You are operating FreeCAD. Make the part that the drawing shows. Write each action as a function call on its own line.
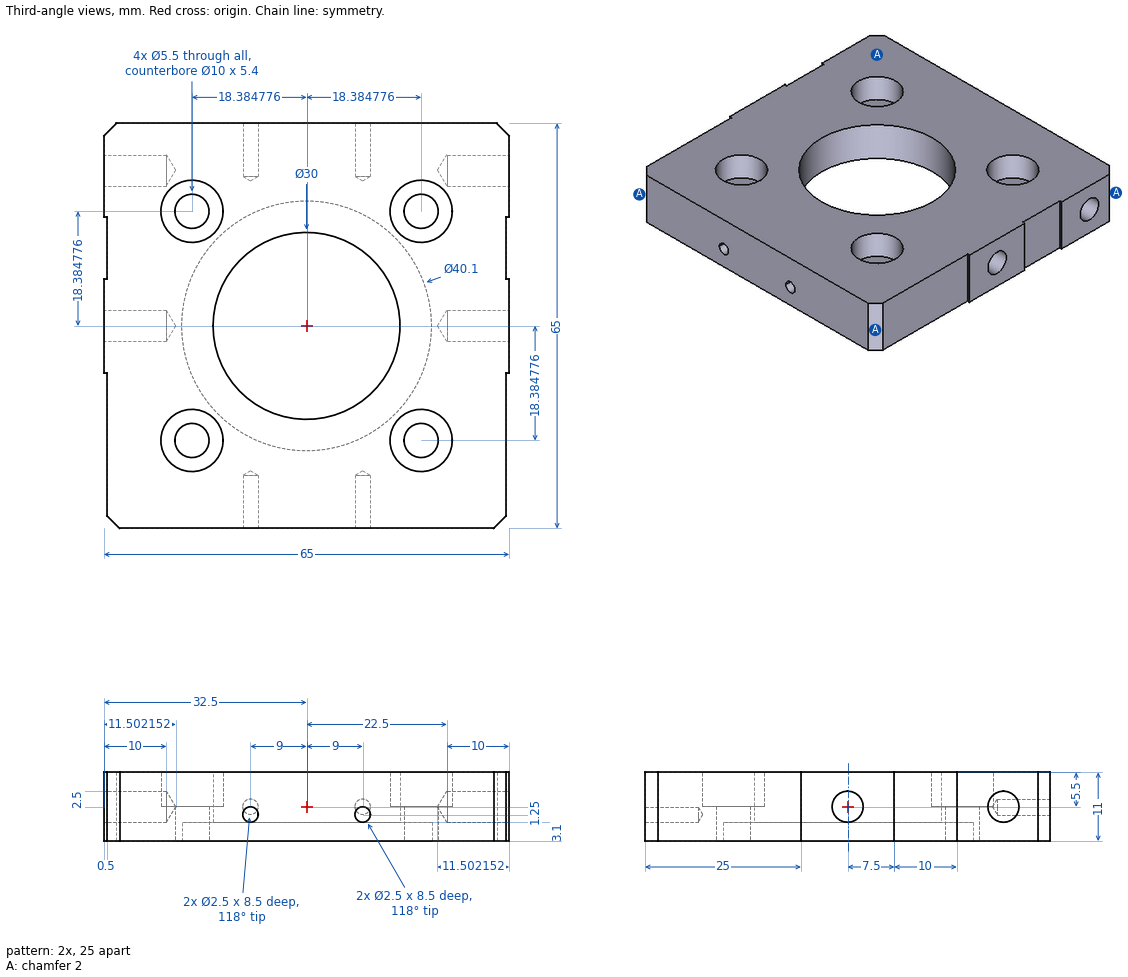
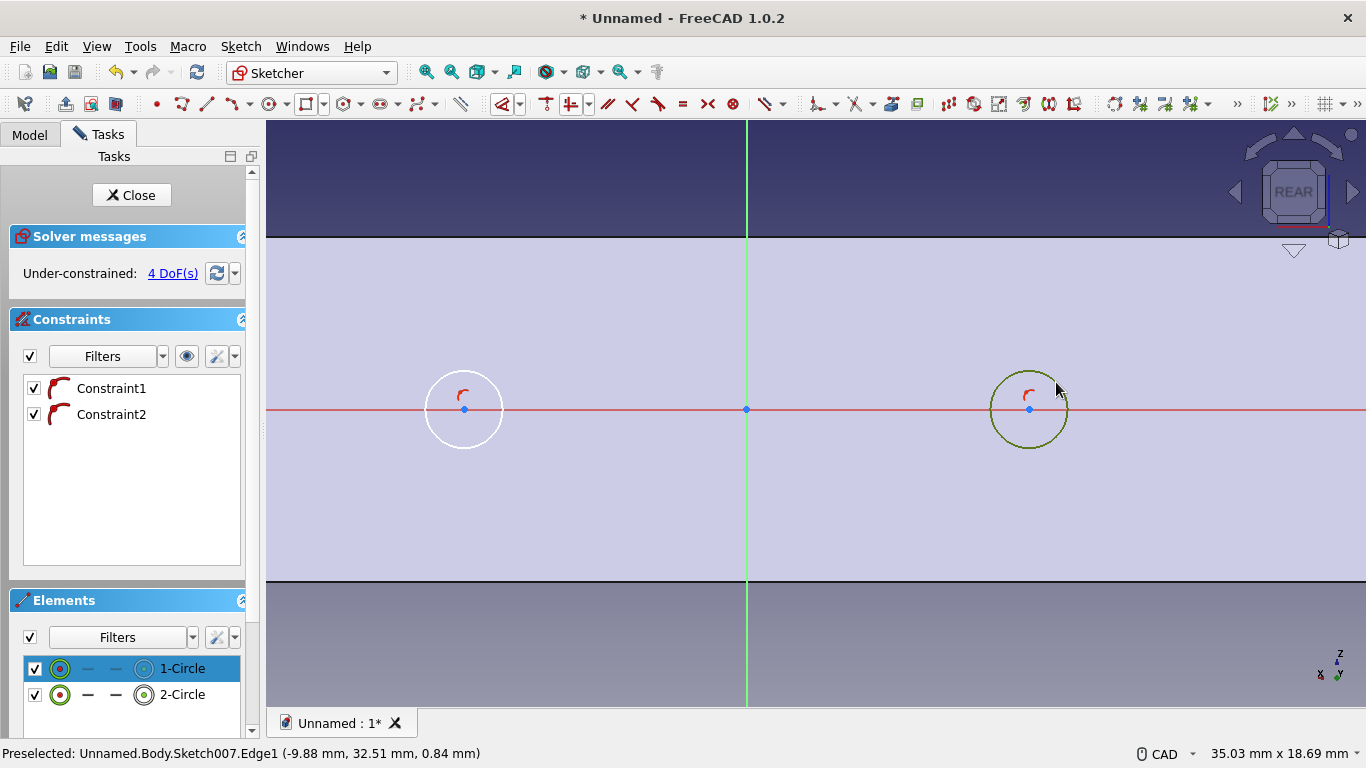
click(491, 382)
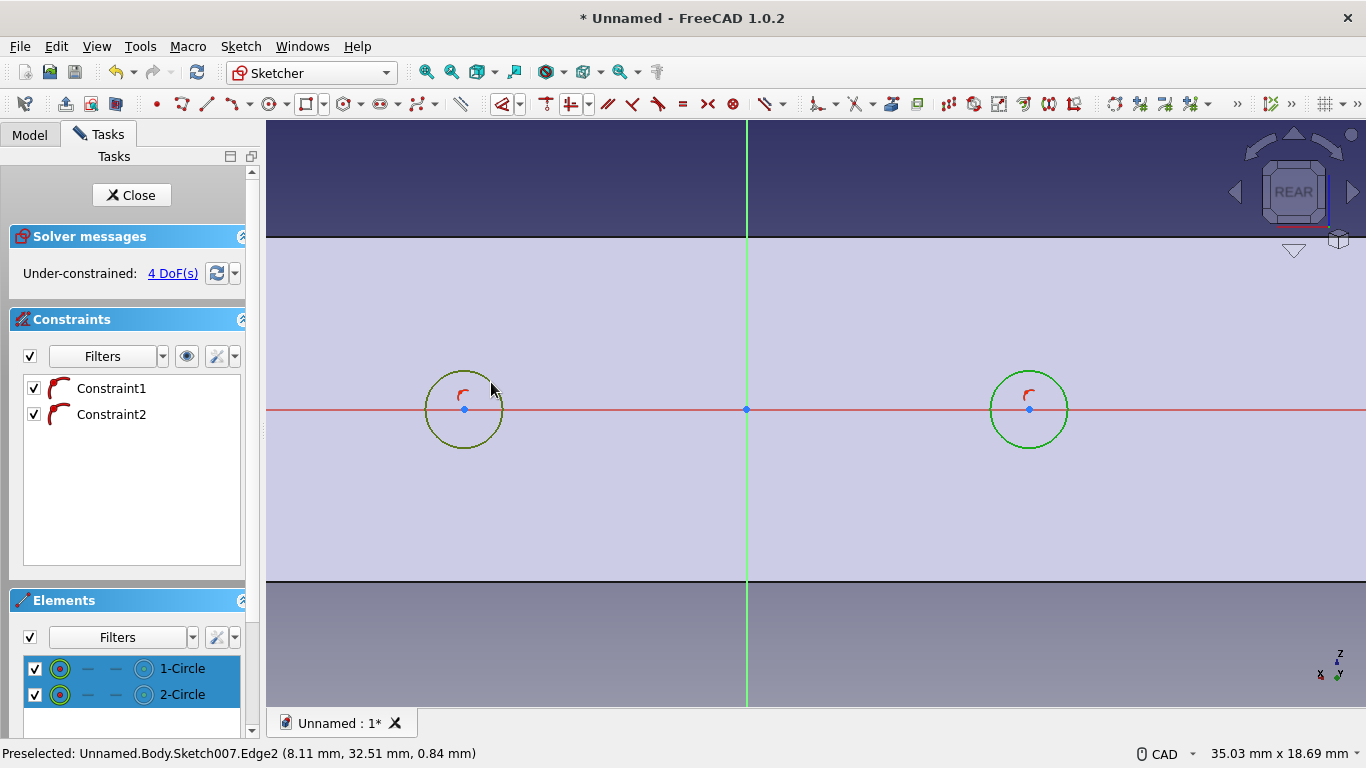
click(683, 104)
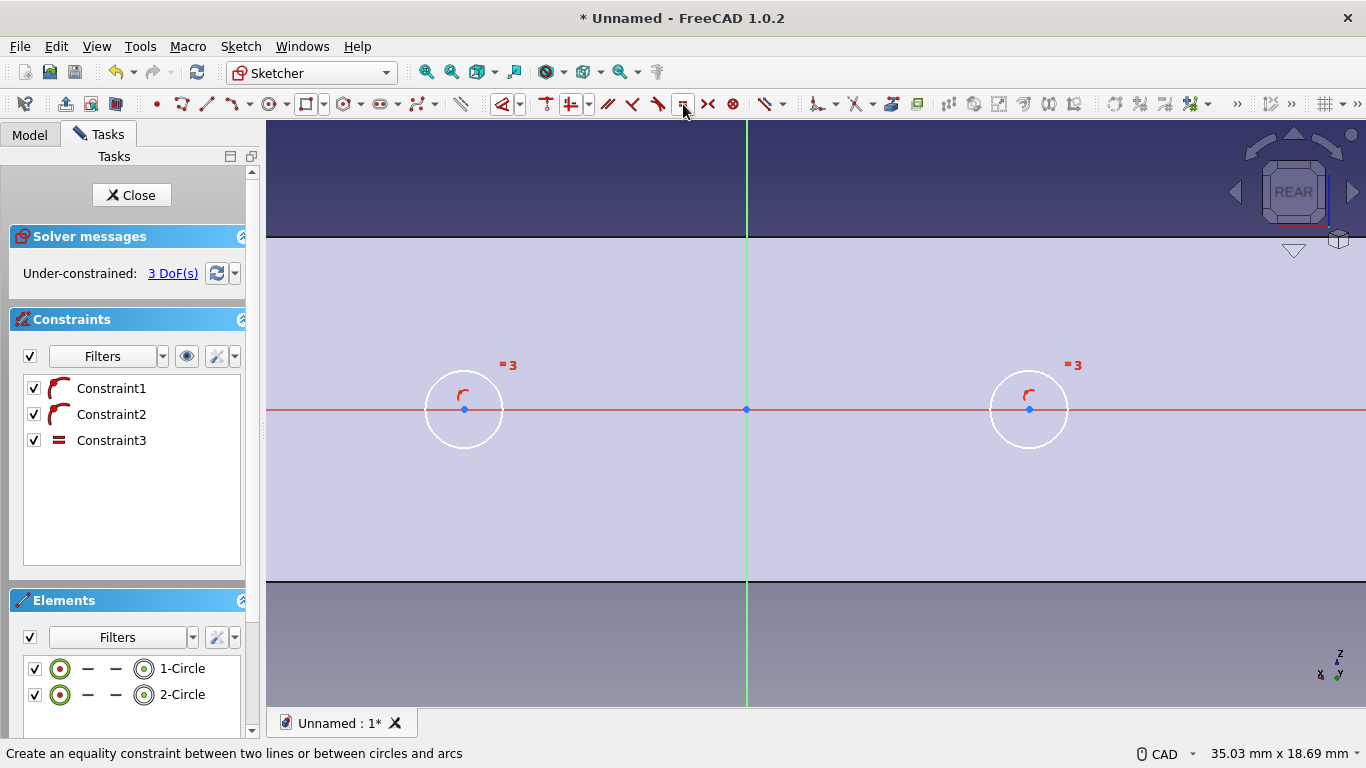
click(1056, 382)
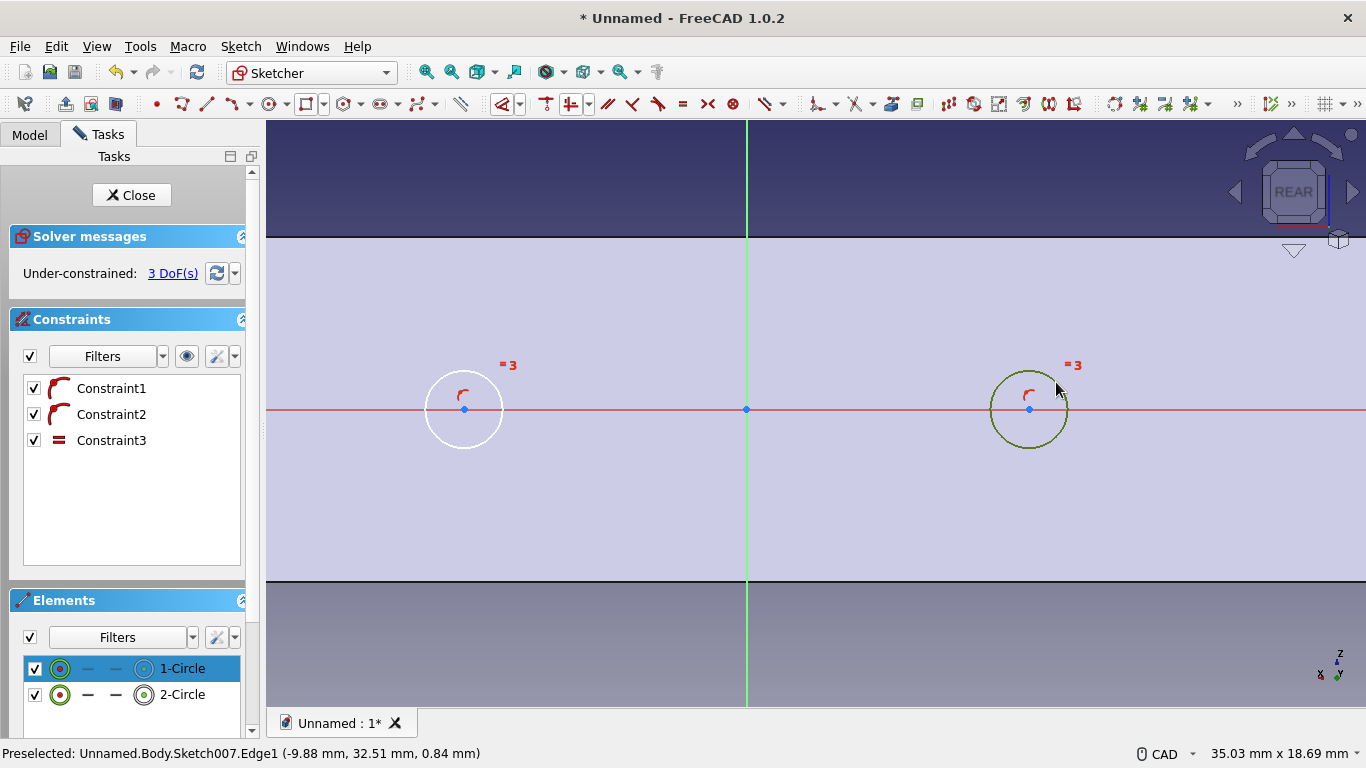
key(k)
key(o)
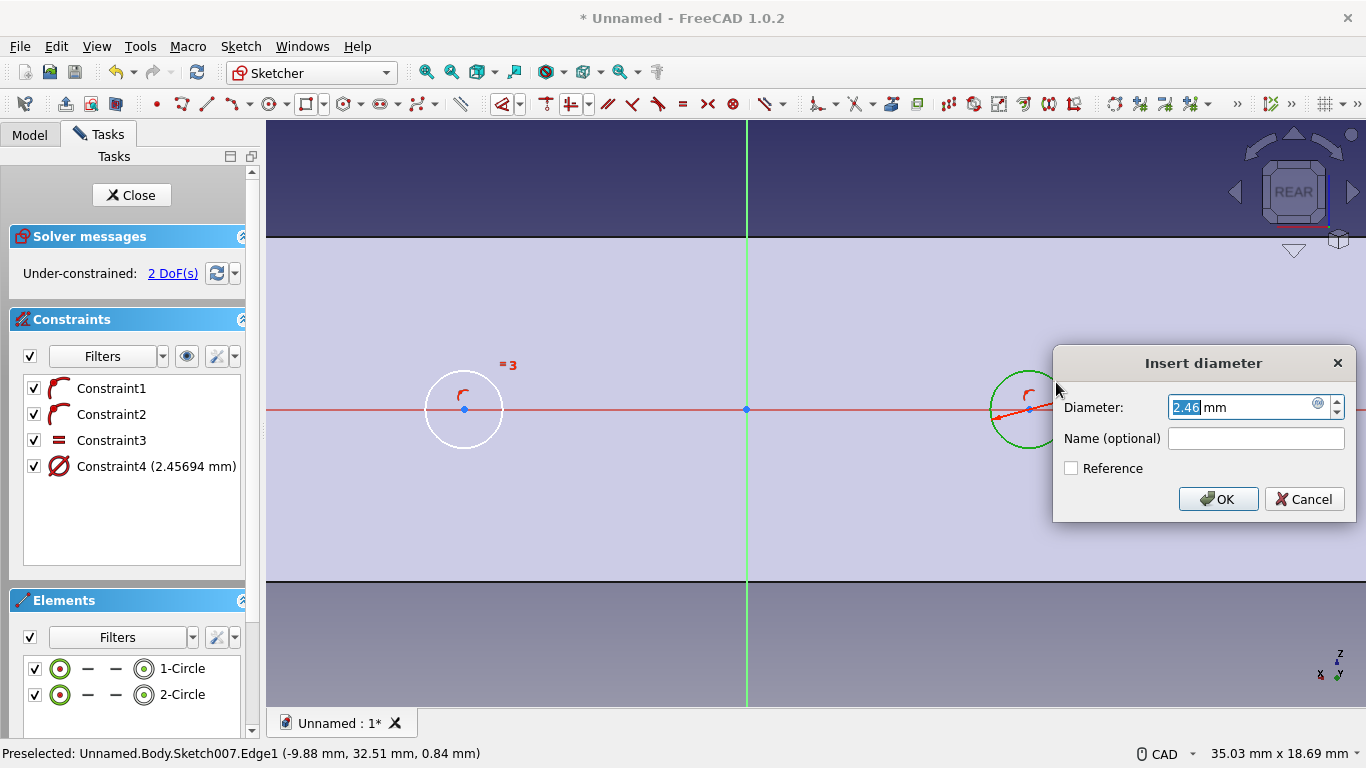
text(2.5)
key(Return)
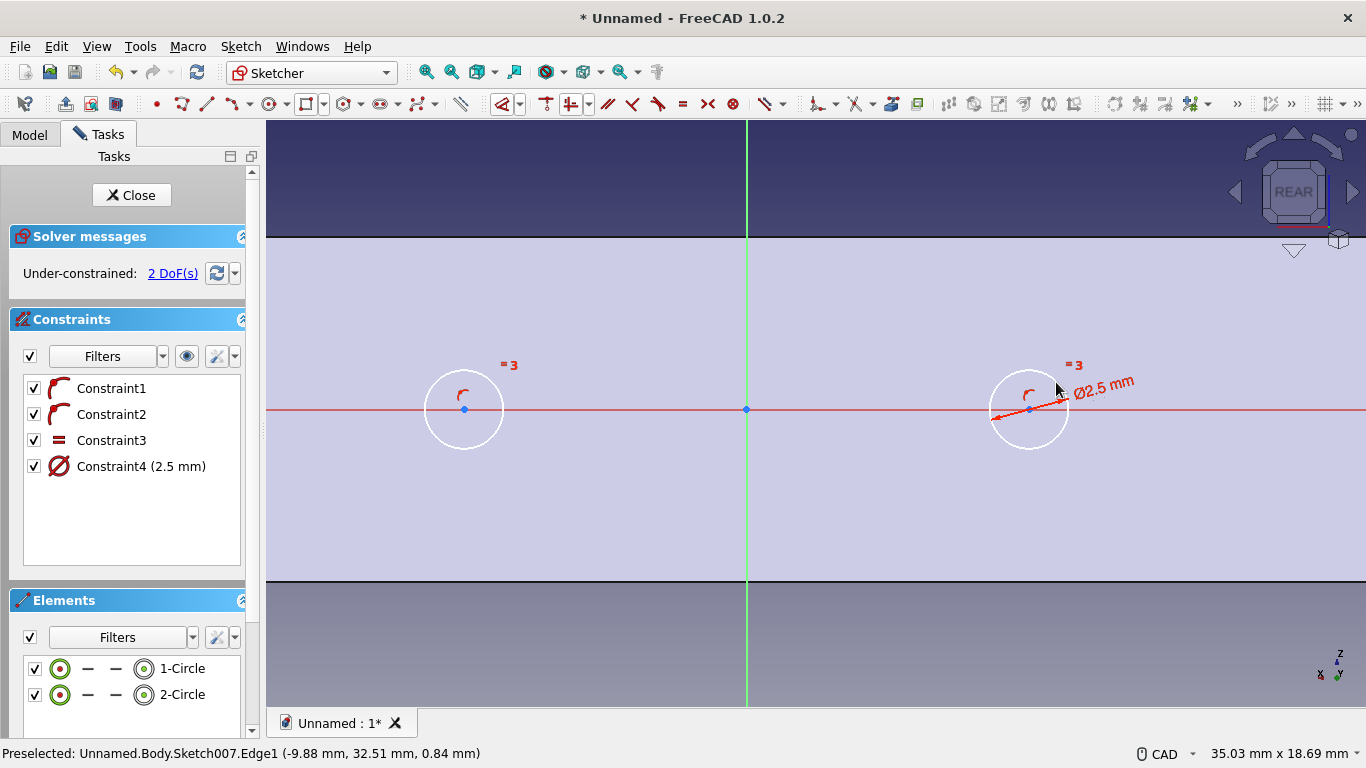
click(1029, 410)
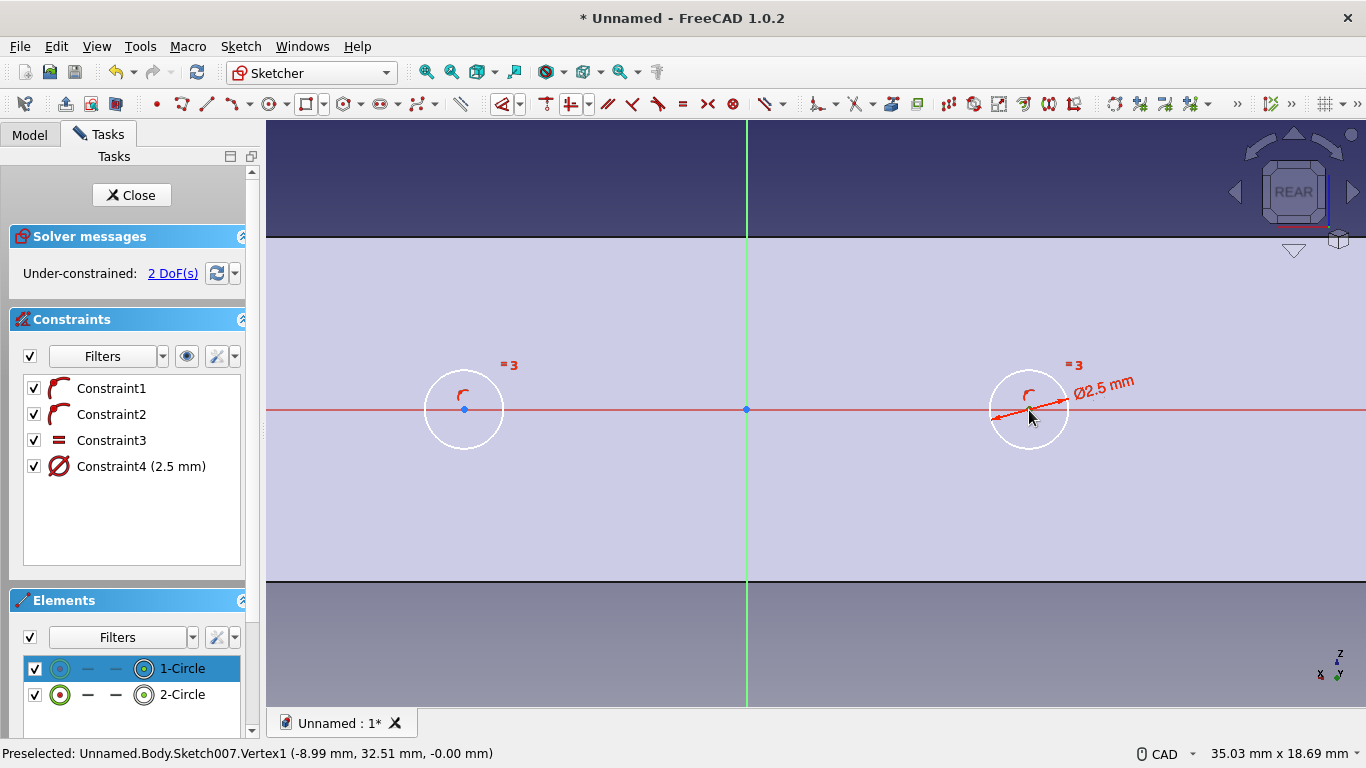
click(520, 104)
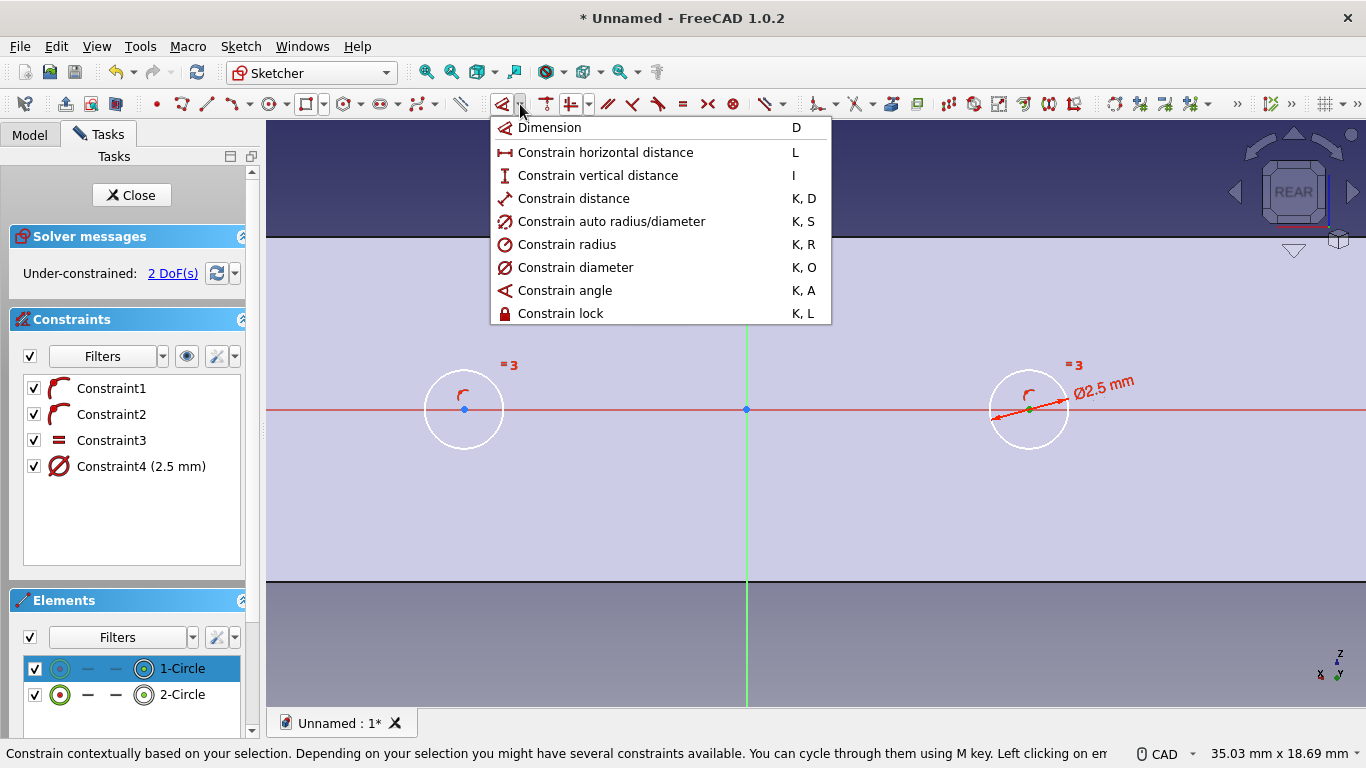
click(661, 152)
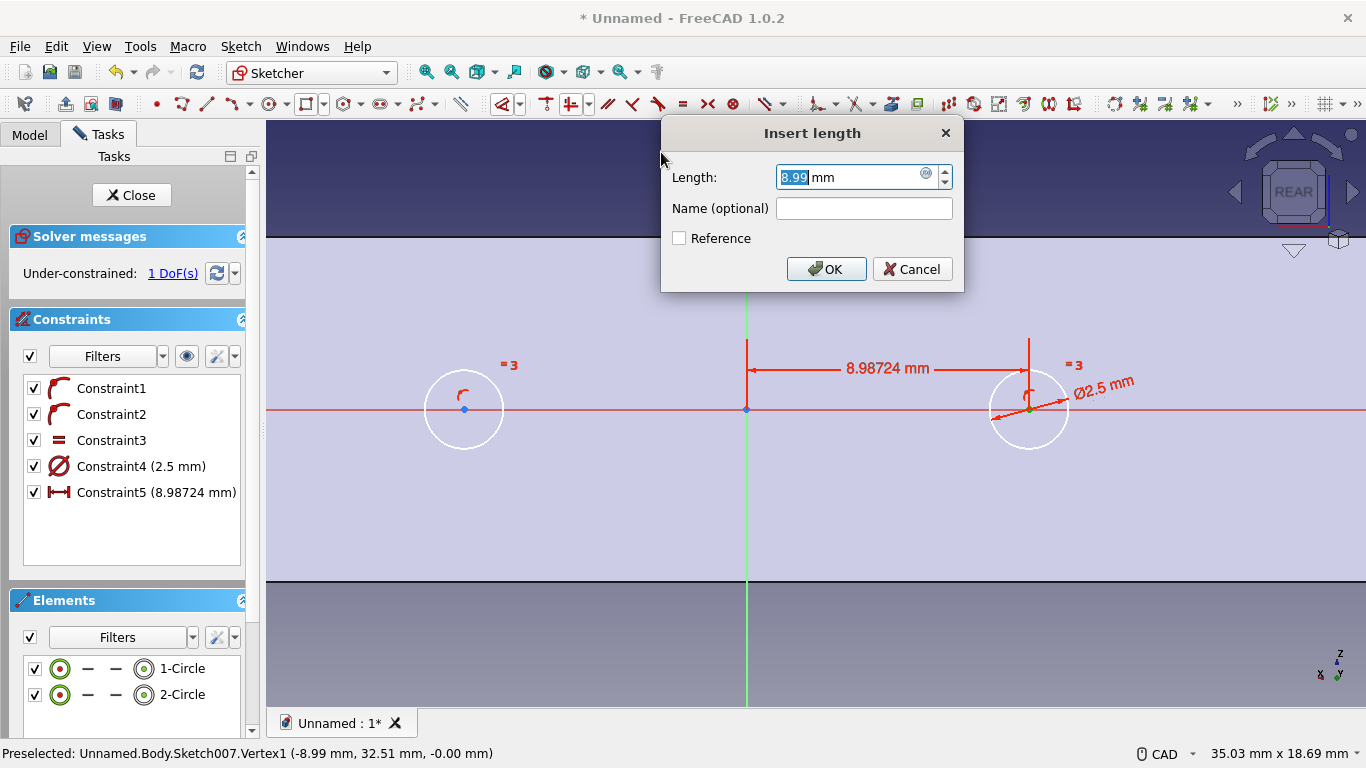
text(9)
key(Return)